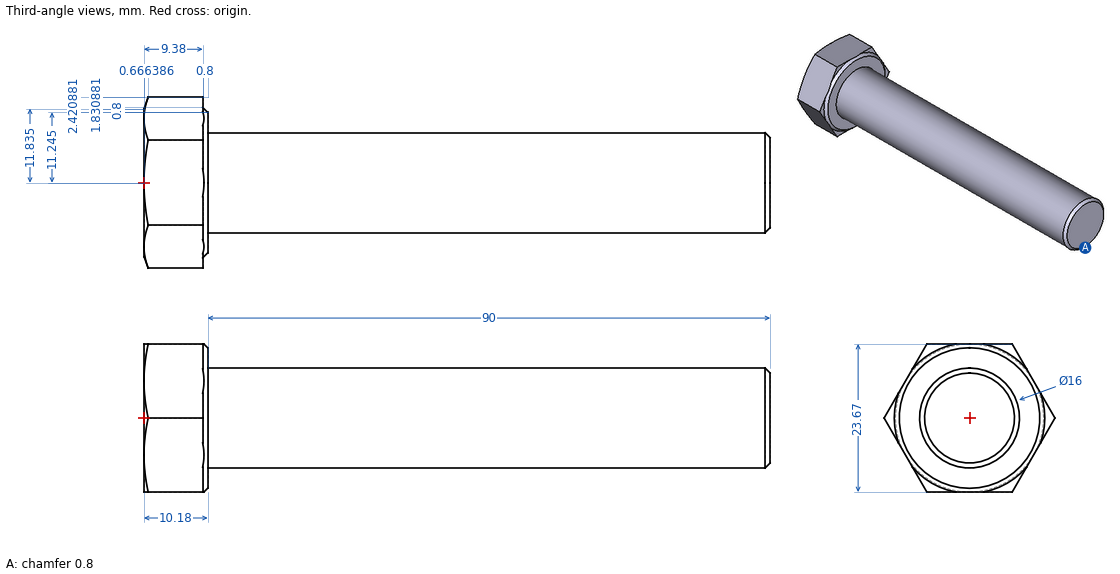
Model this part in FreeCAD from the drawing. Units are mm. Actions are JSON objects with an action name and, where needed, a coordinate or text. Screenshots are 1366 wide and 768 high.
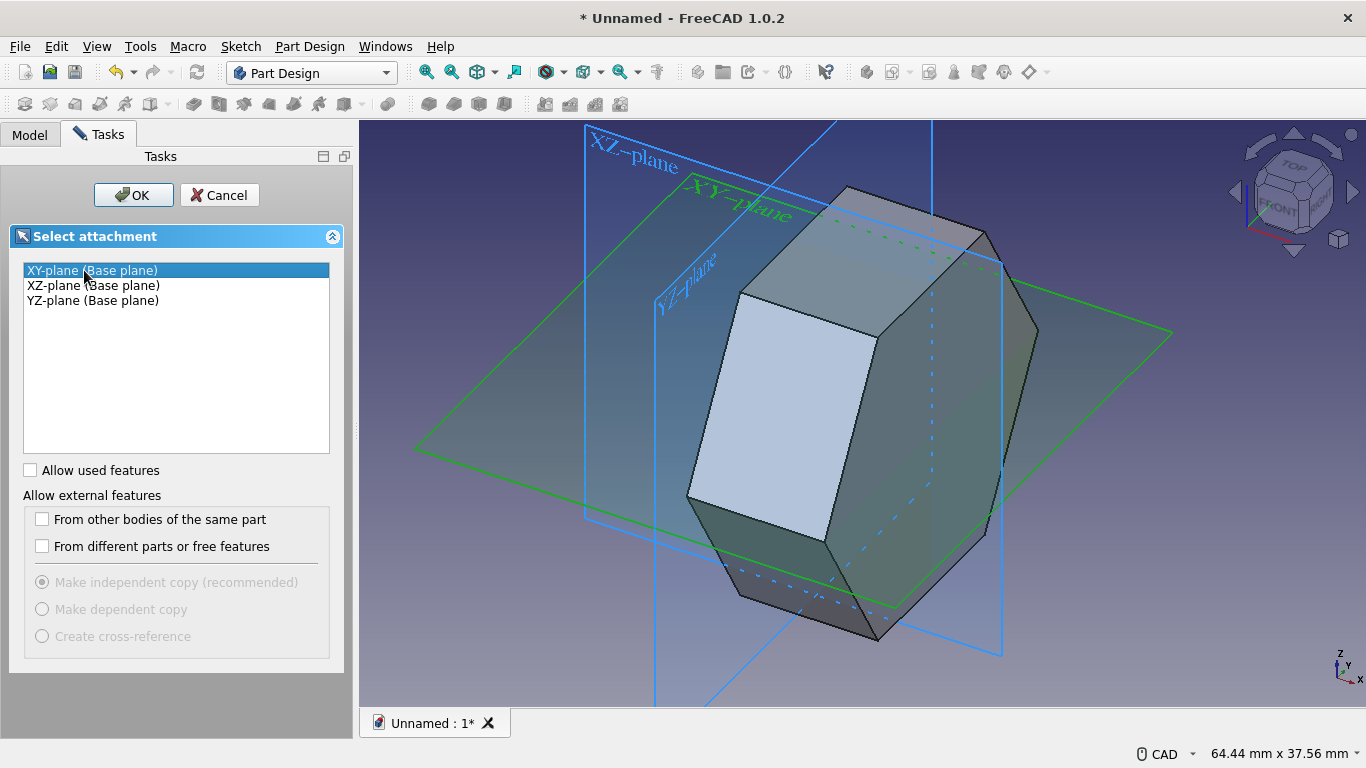
{"action": "left_click", "coordinate": [134, 195]}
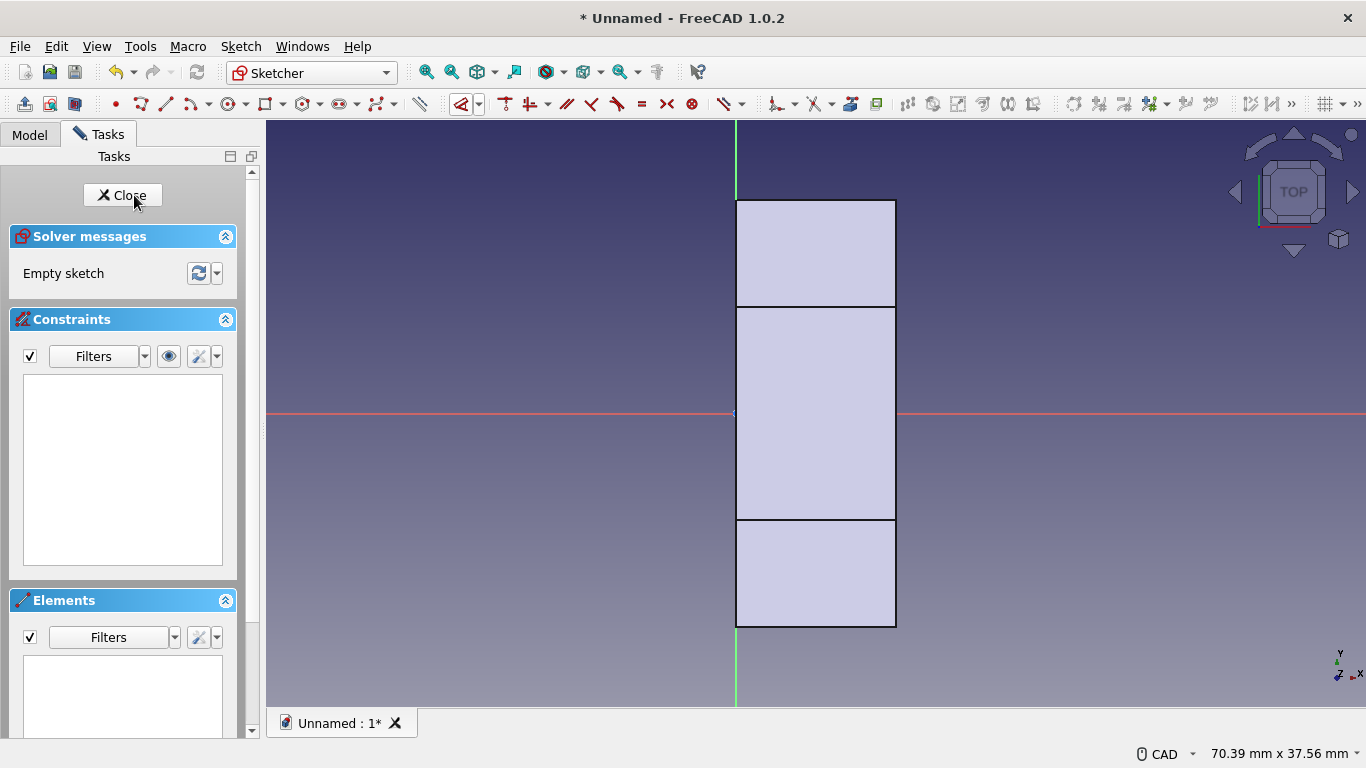
{"action": "key", "text": "q s"}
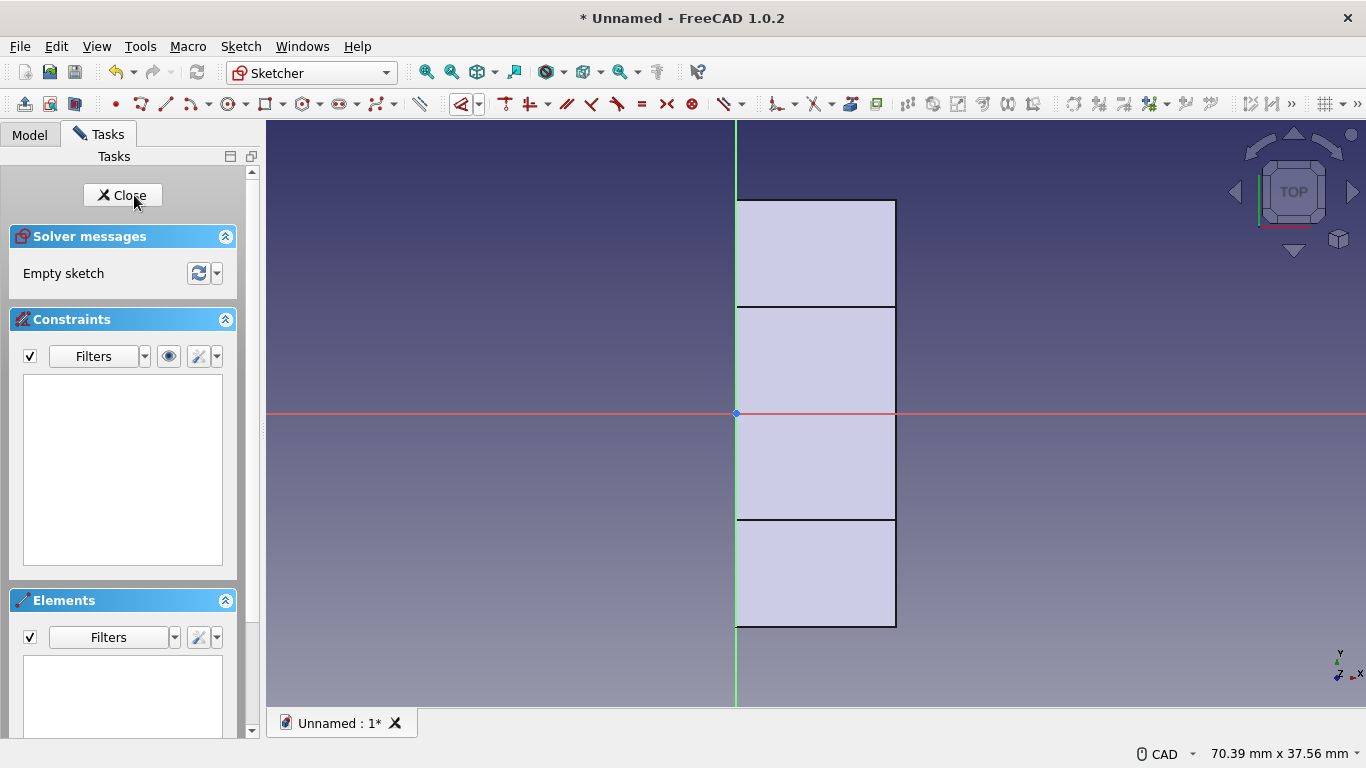
{"action": "scroll", "coordinate": [907, 195], "scroll_direction": "up", "scroll_amount": 11}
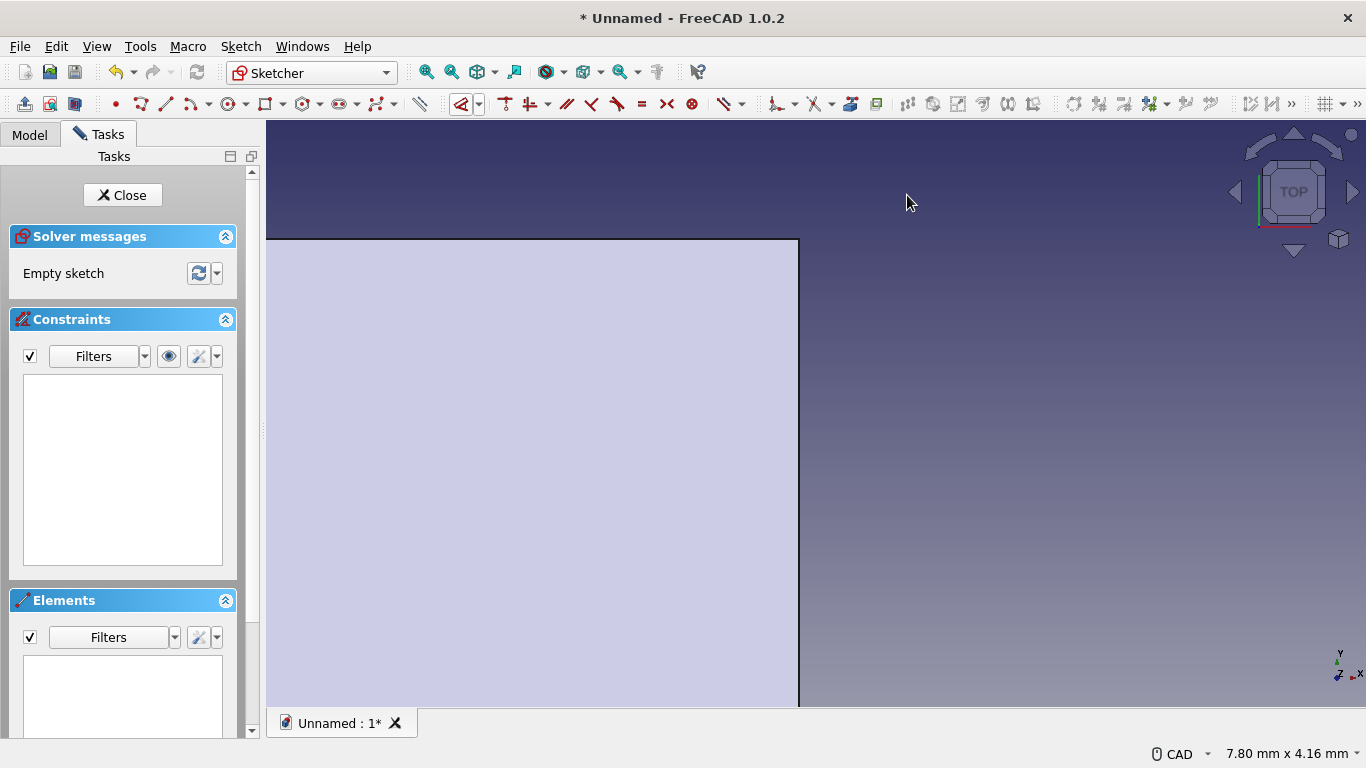
{"action": "key", "text": "g m"}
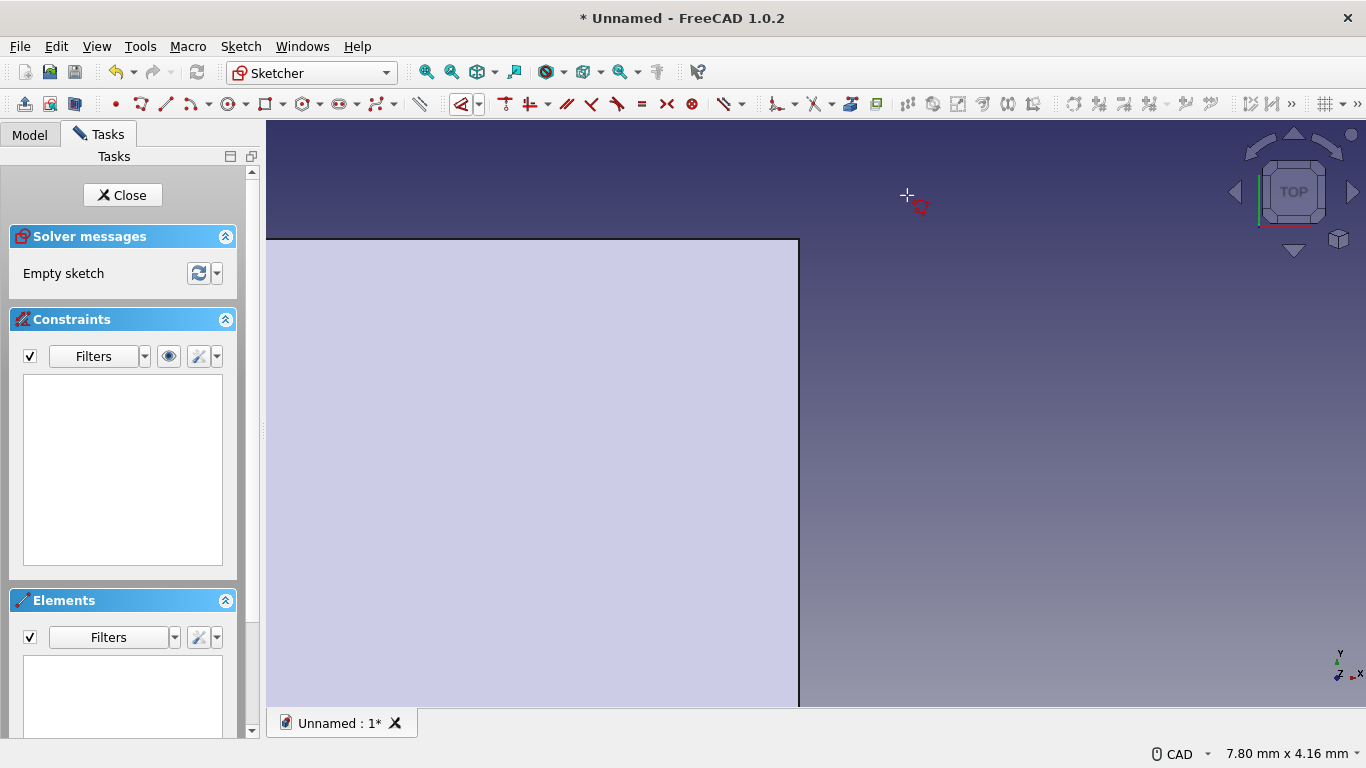
{"action": "left_click", "coordinate": [799, 580]}
{"action": "left_click", "coordinate": [799, 239]}
{"action": "left_click", "coordinate": [686, 239]}
{"action": "left_click", "coordinate": [686, 467]}
{"action": "left_click", "coordinate": [799, 581]}
{"action": "key", "text": "Escape"}
{"action": "key", "text": "Escape"}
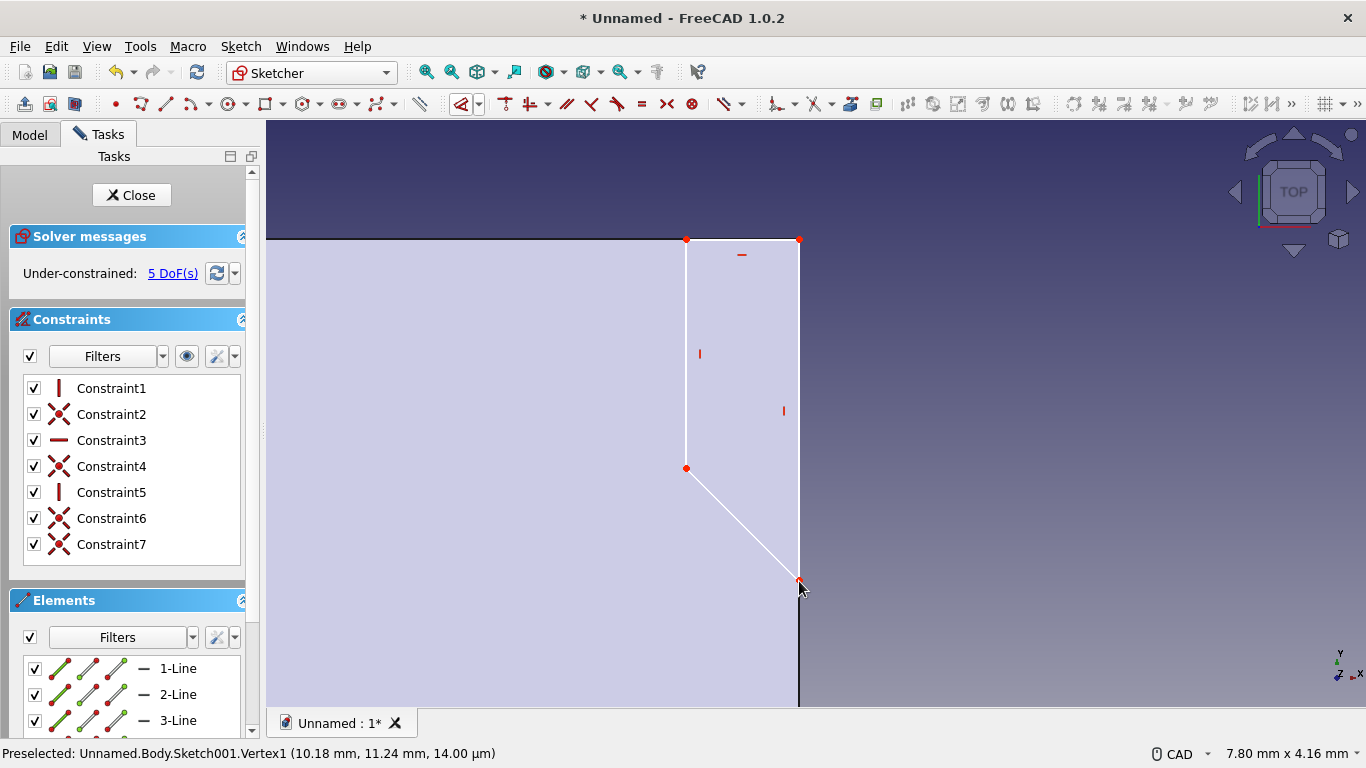
{"action": "left_click", "coordinate": [765, 240]}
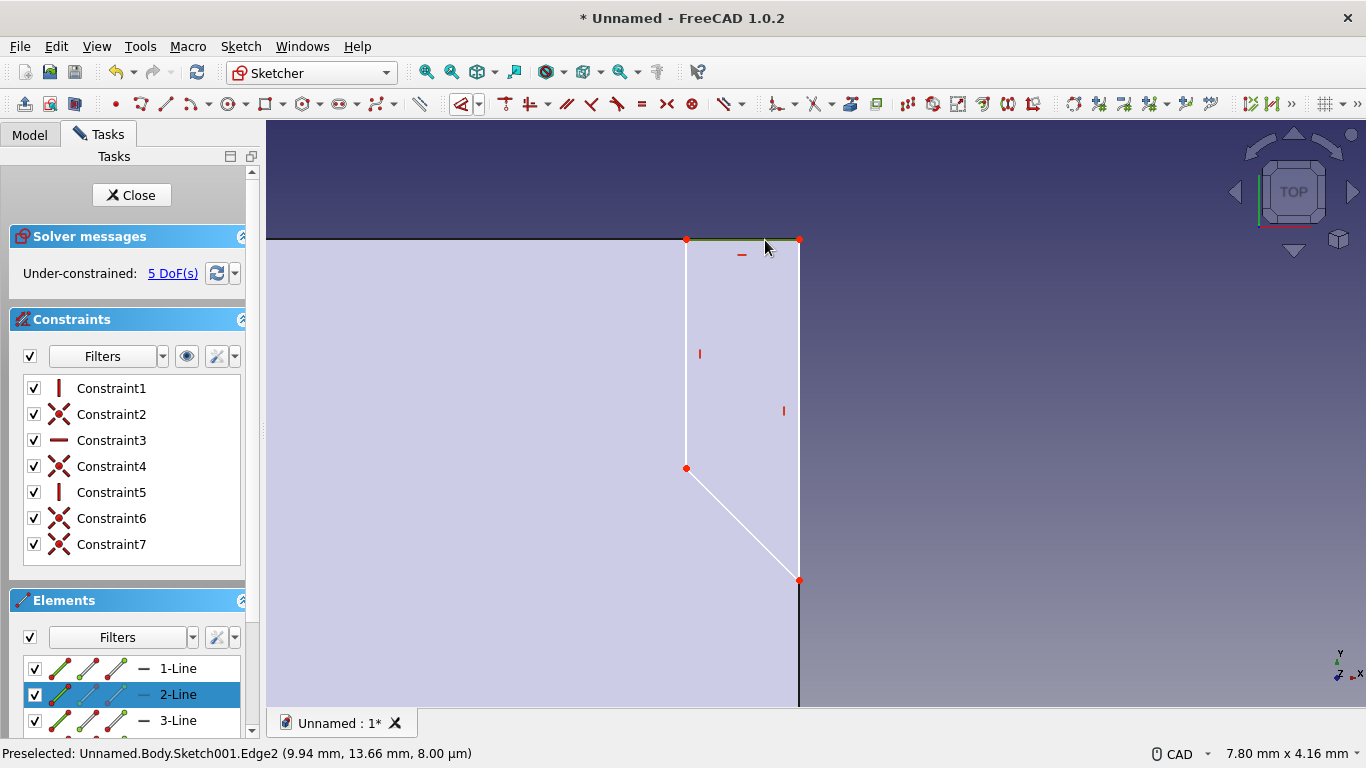
{"action": "key", "text": "l"}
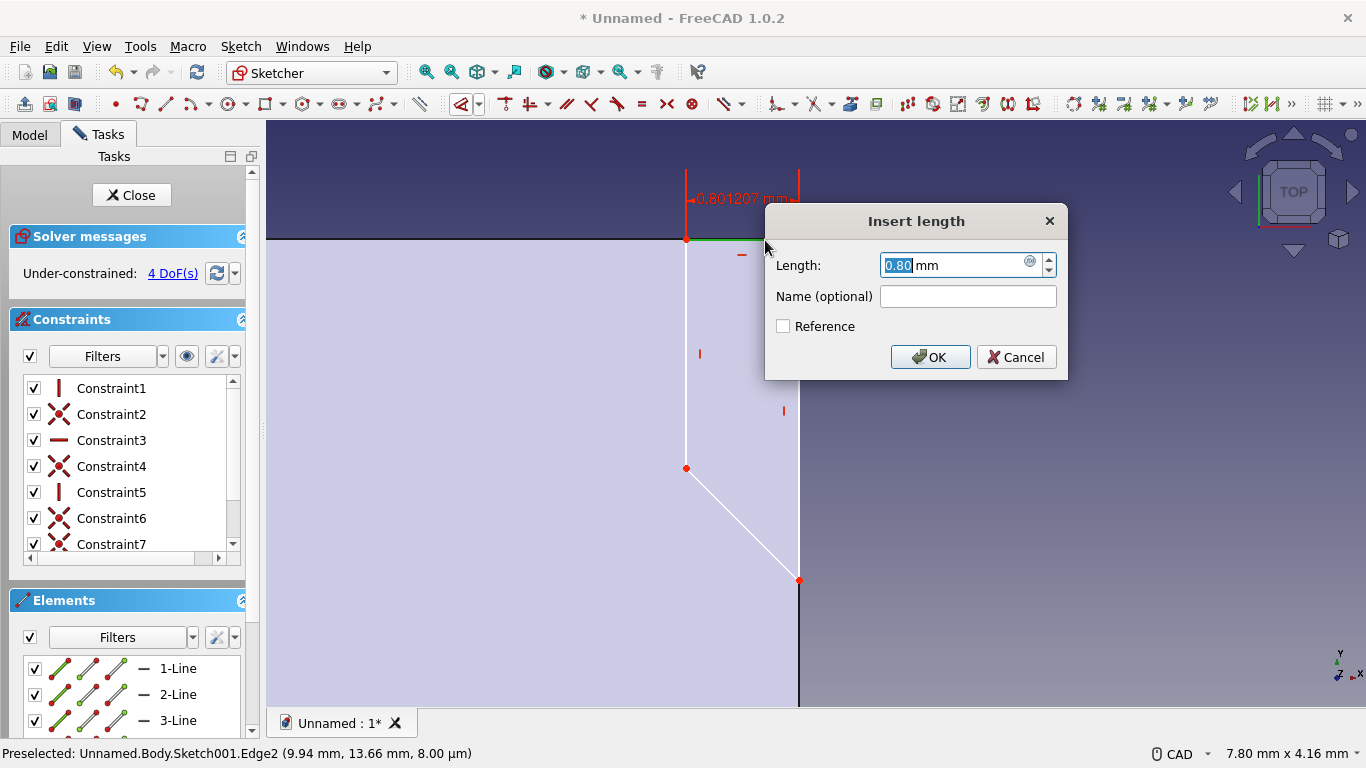
{"action": "type", "text": "0.8"}
{"action": "key", "text": "Return"}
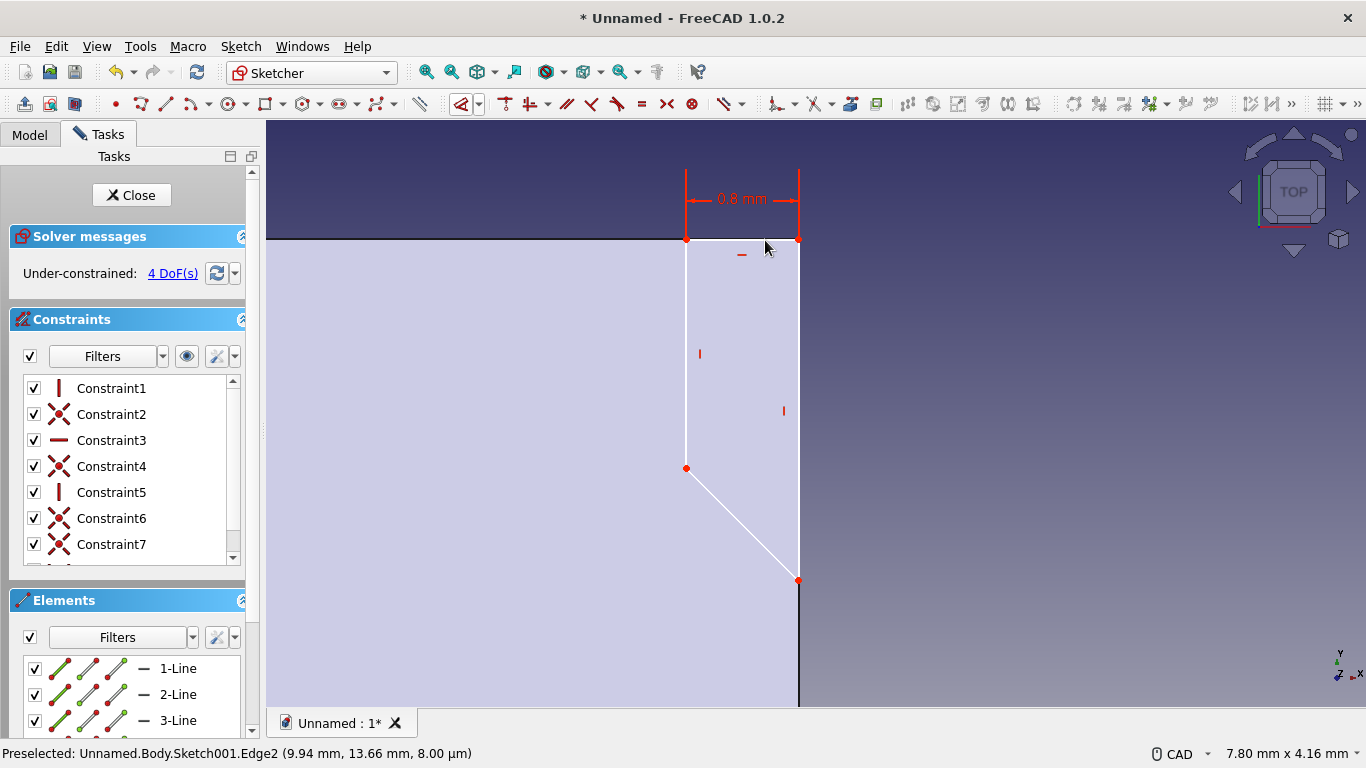
{"action": "left_click", "coordinate": [720, 502]}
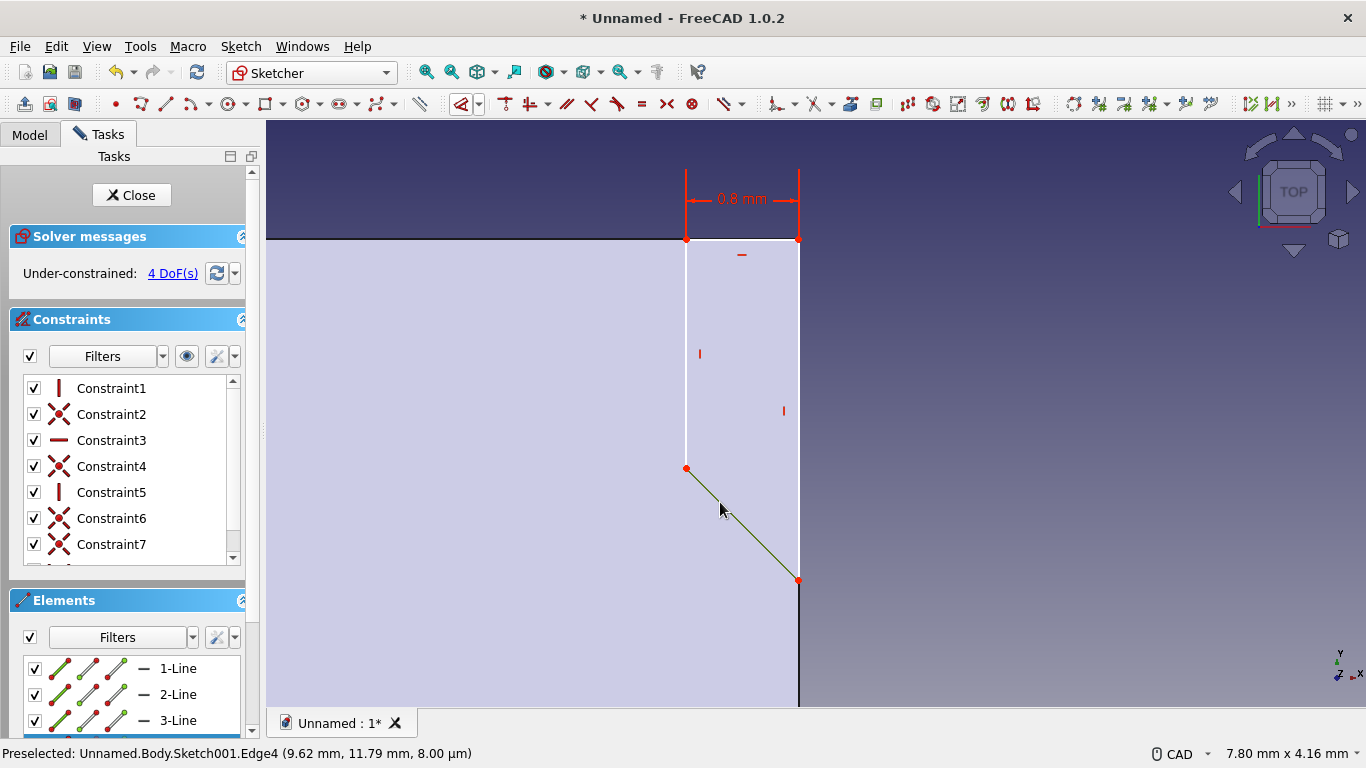
{"action": "key", "text": "i"}